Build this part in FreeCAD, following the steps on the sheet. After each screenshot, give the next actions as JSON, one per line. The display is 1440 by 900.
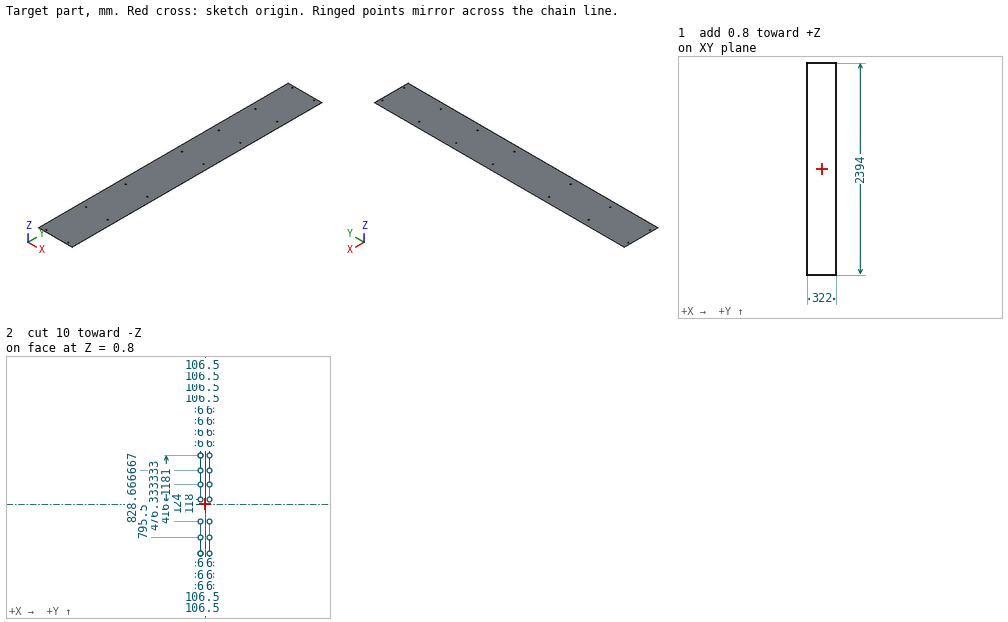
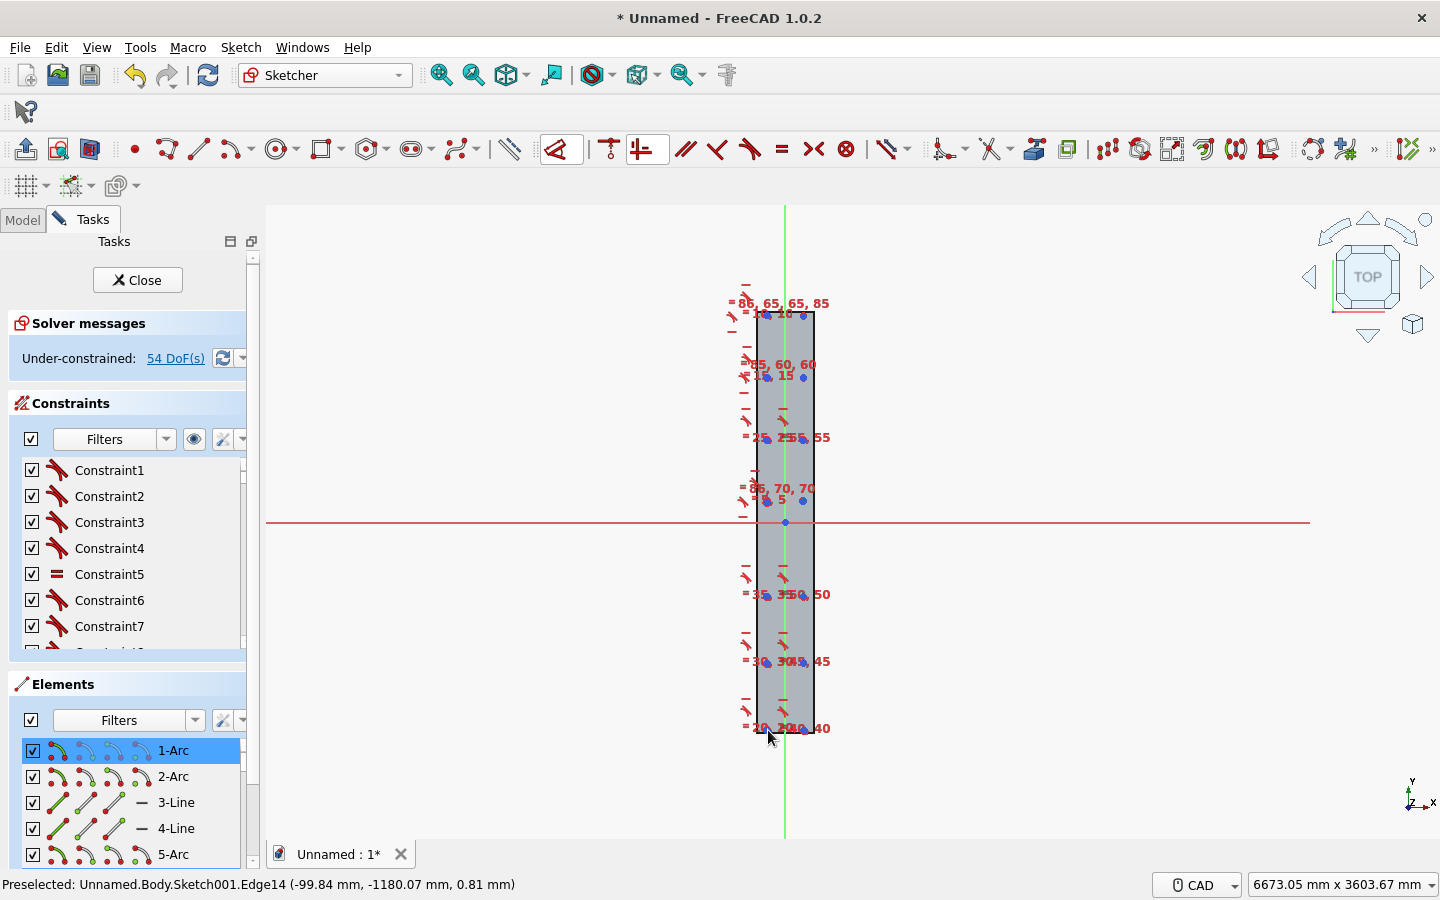
{"action": "scroll", "coordinate": [768, 440], "scroll_direction": "up", "scroll_amount": 14}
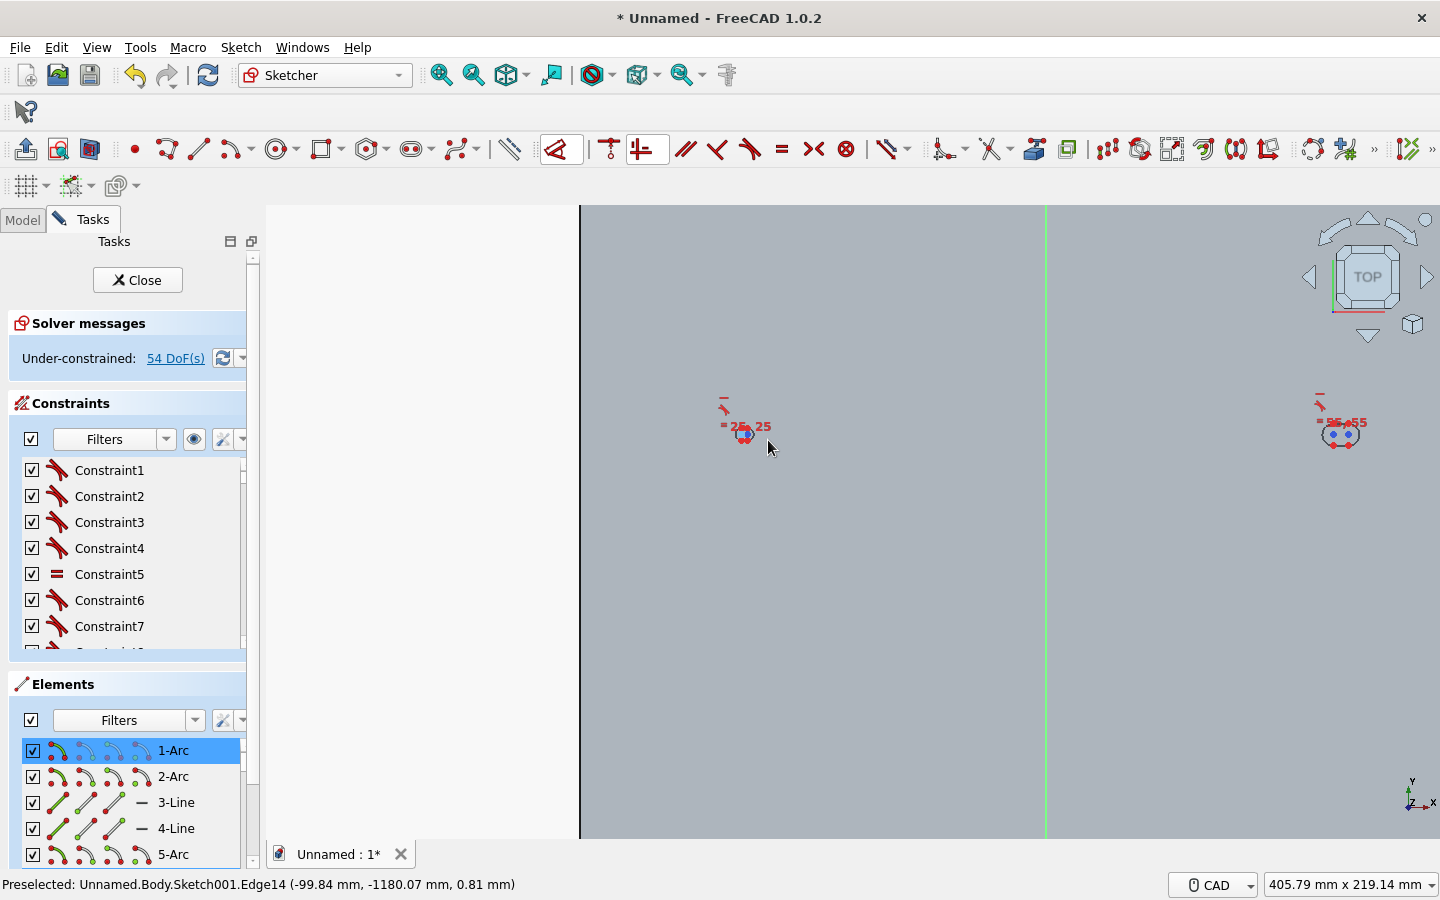
{"action": "left_click", "coordinate": [754, 434]}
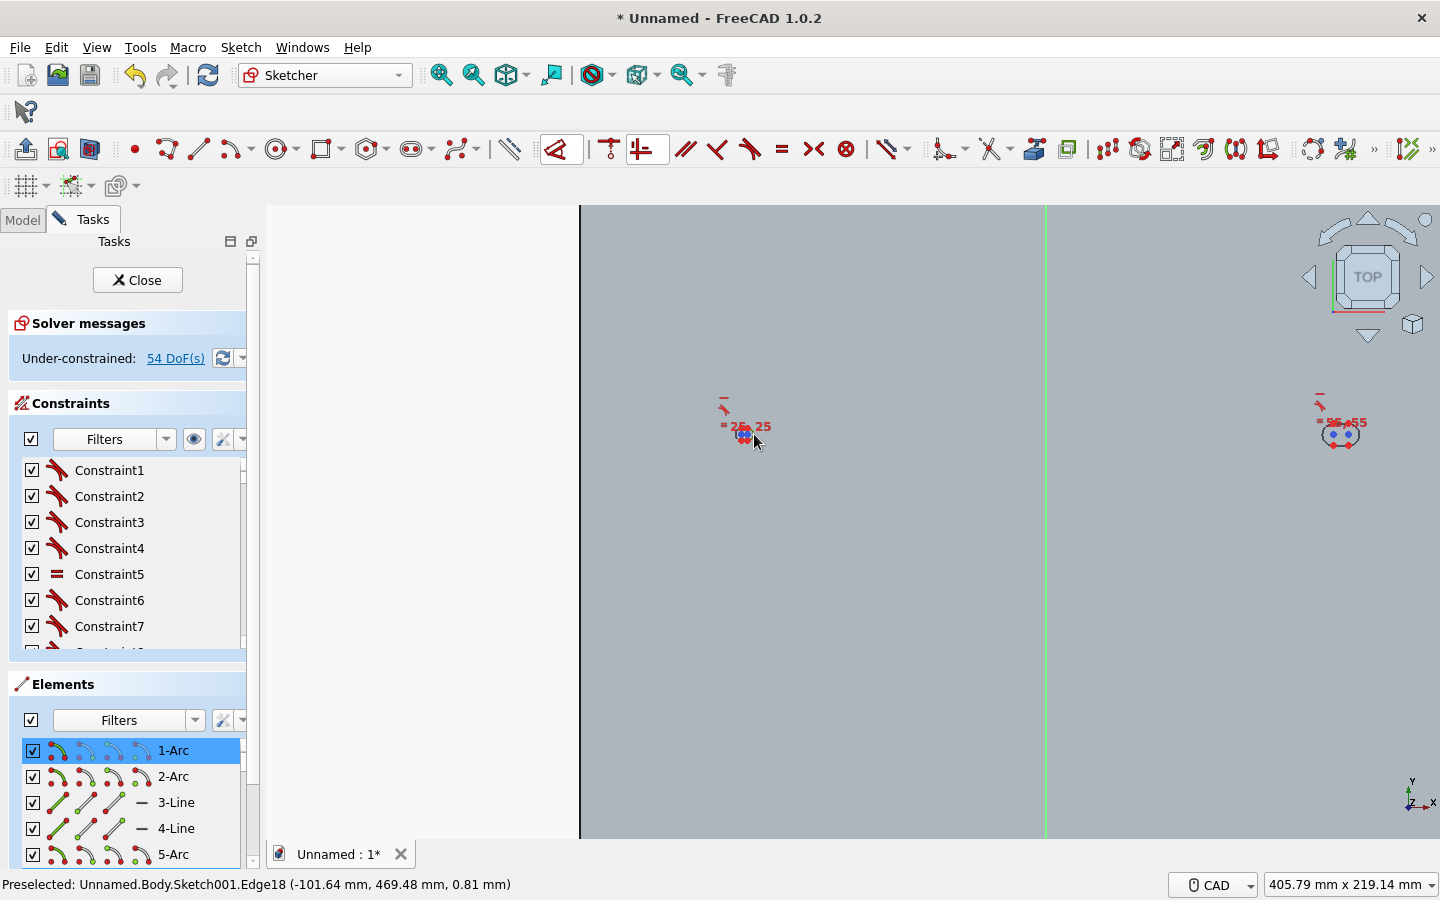
{"action": "scroll", "coordinate": [768, 439], "scroll_direction": "down", "scroll_amount": 14}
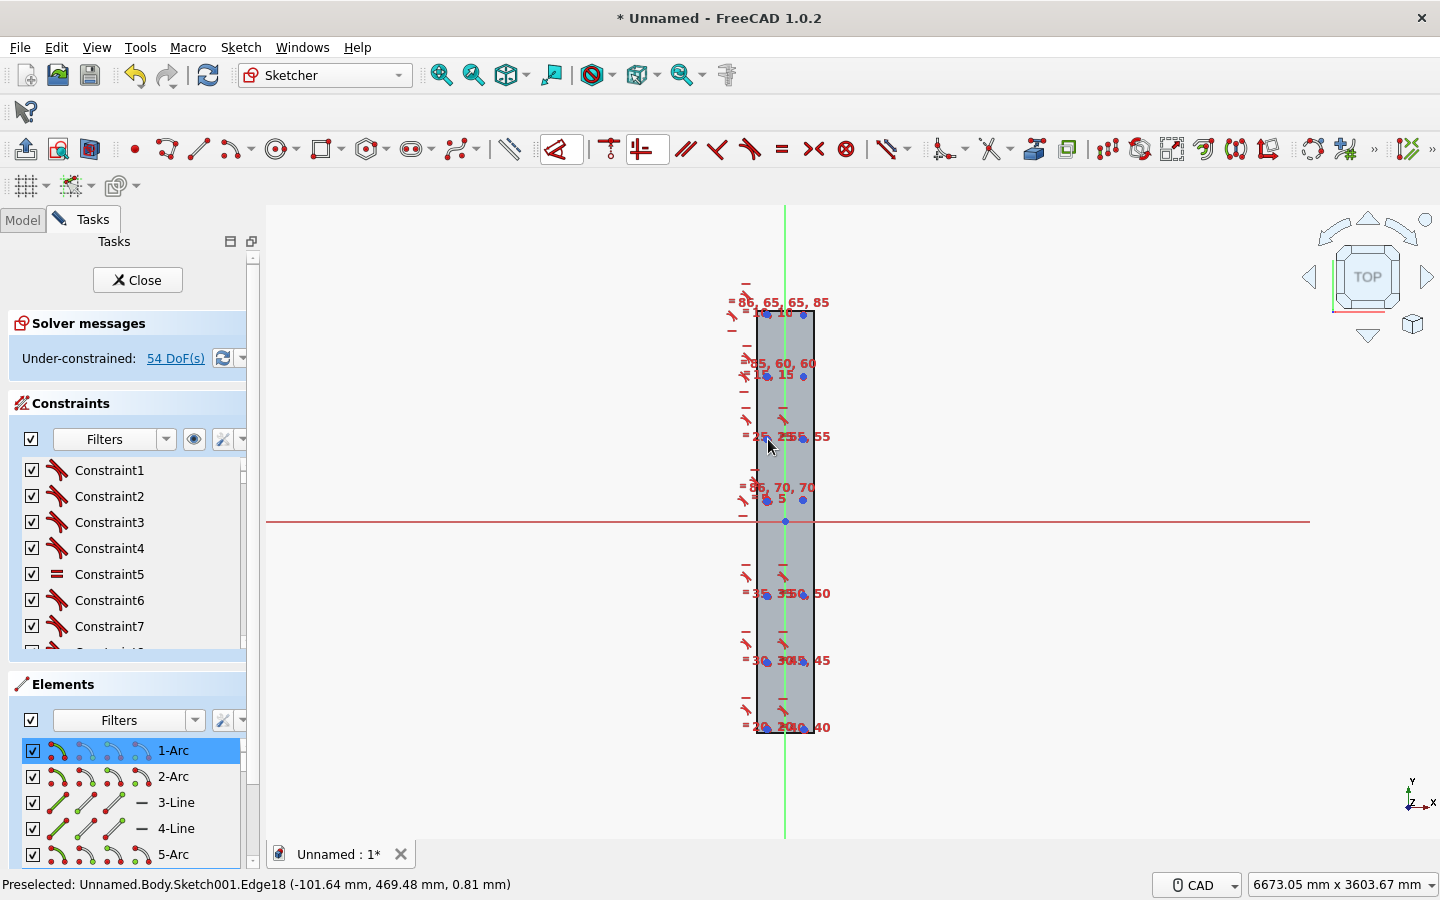
{"action": "scroll", "coordinate": [768, 663], "scroll_direction": "up", "scroll_amount": 14}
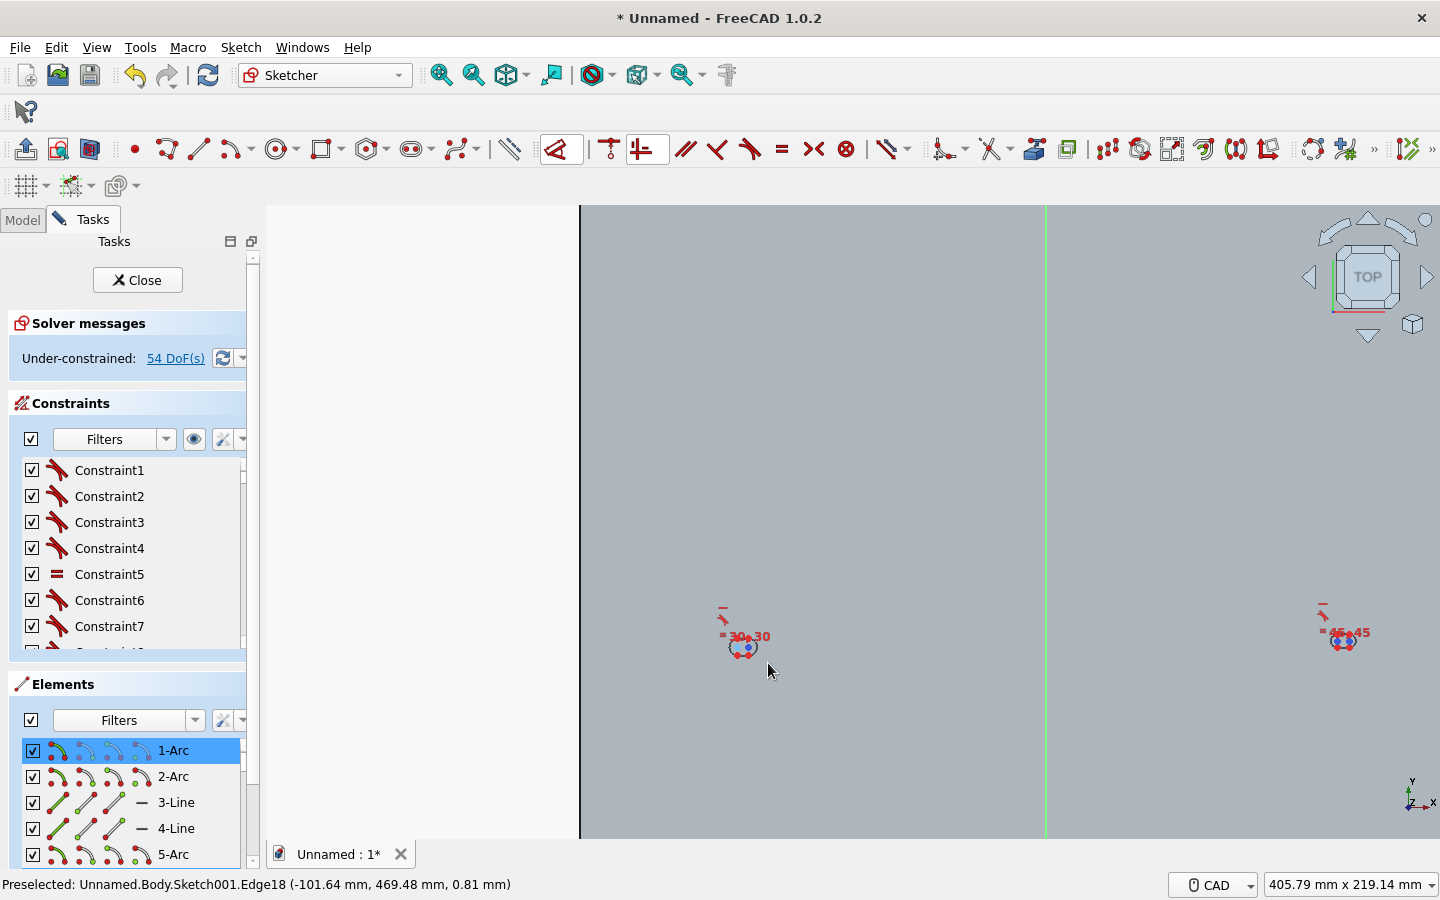
{"action": "left_click", "coordinate": [757, 647]}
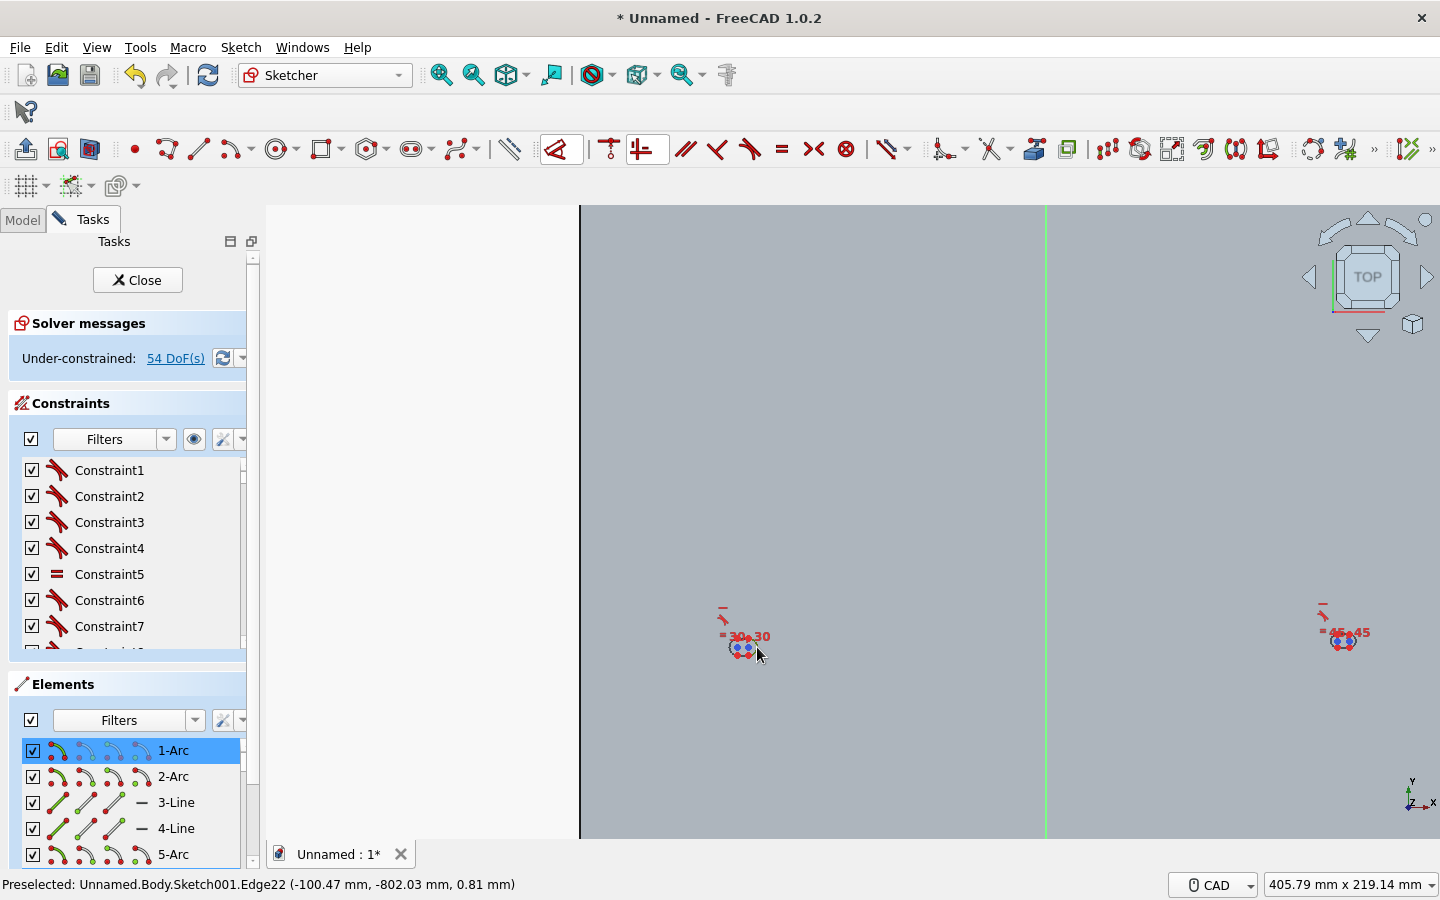
{"action": "scroll", "coordinate": [768, 664], "scroll_direction": "down", "scroll_amount": 14}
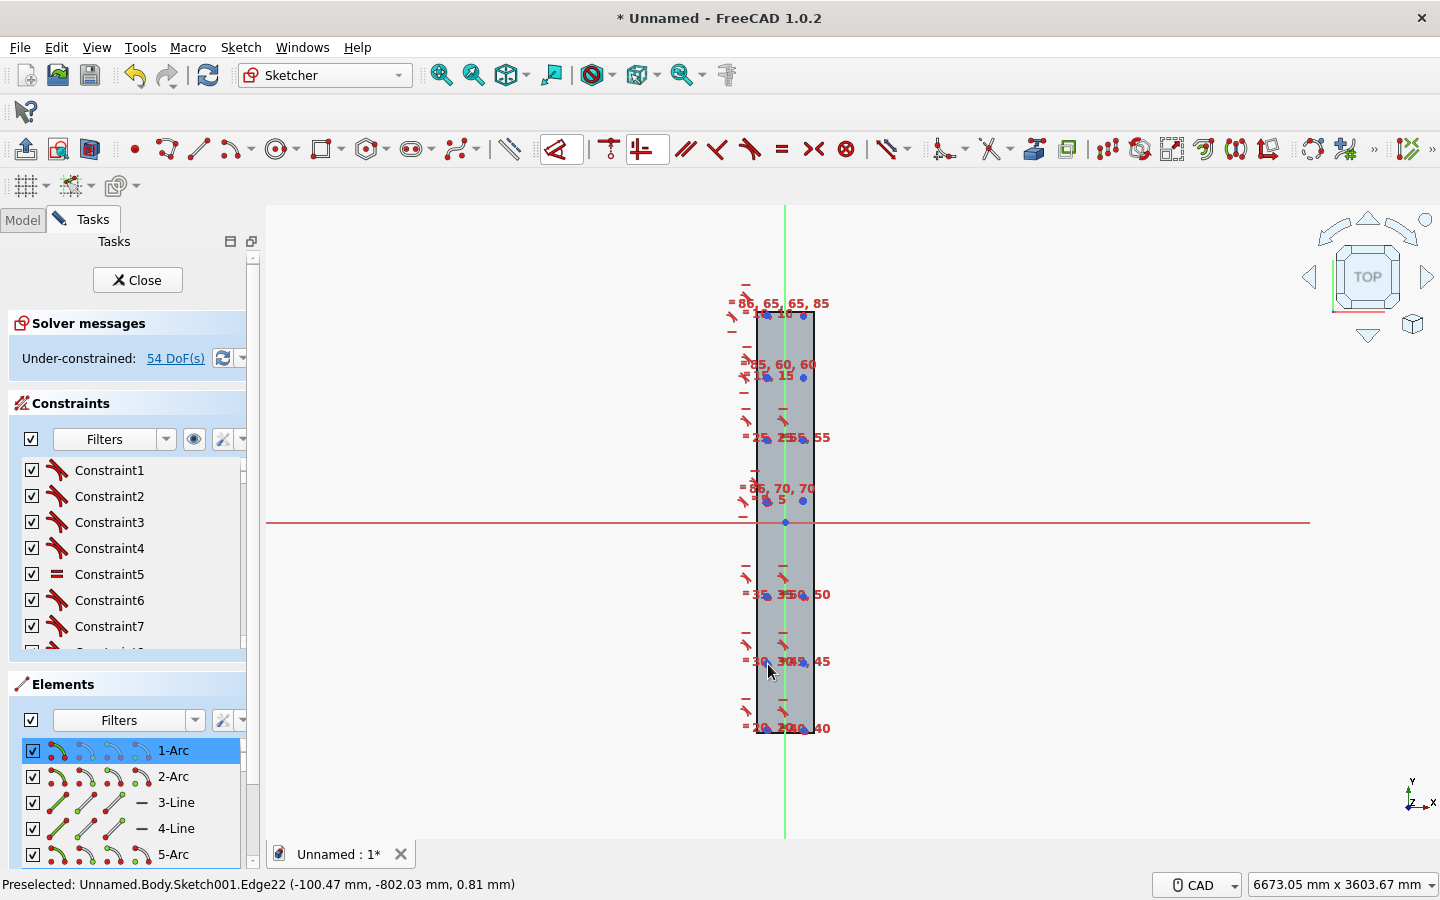
{"action": "scroll", "coordinate": [767, 597], "scroll_direction": "up", "scroll_amount": 14}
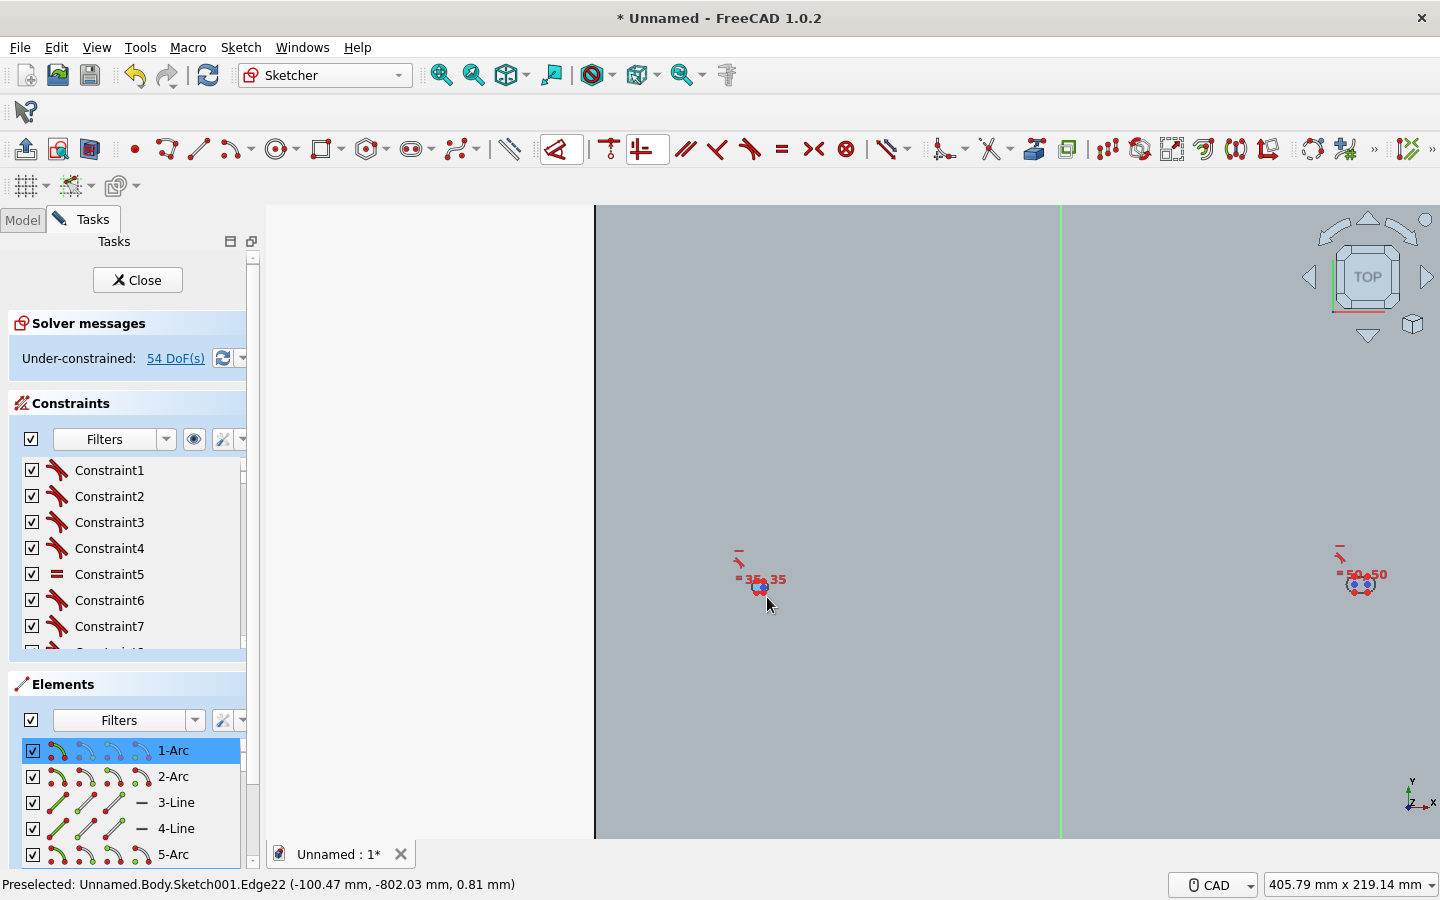
{"action": "scroll", "coordinate": [768, 587], "scroll_direction": "up", "scroll_amount": 4}